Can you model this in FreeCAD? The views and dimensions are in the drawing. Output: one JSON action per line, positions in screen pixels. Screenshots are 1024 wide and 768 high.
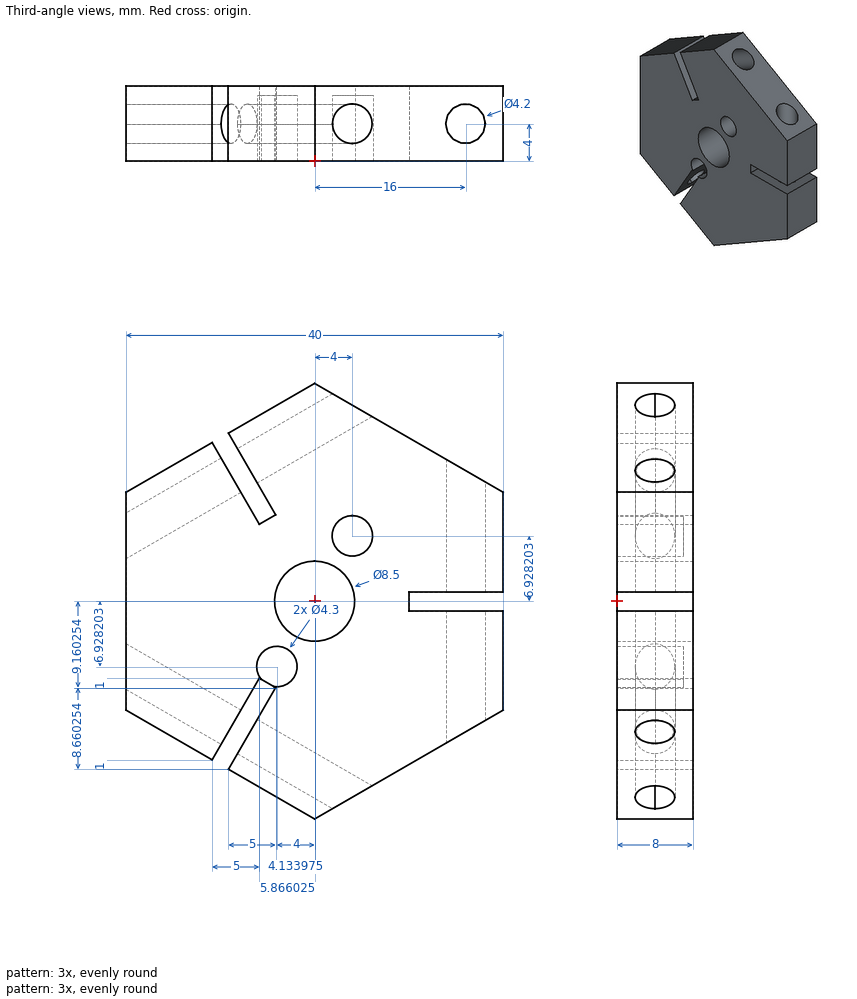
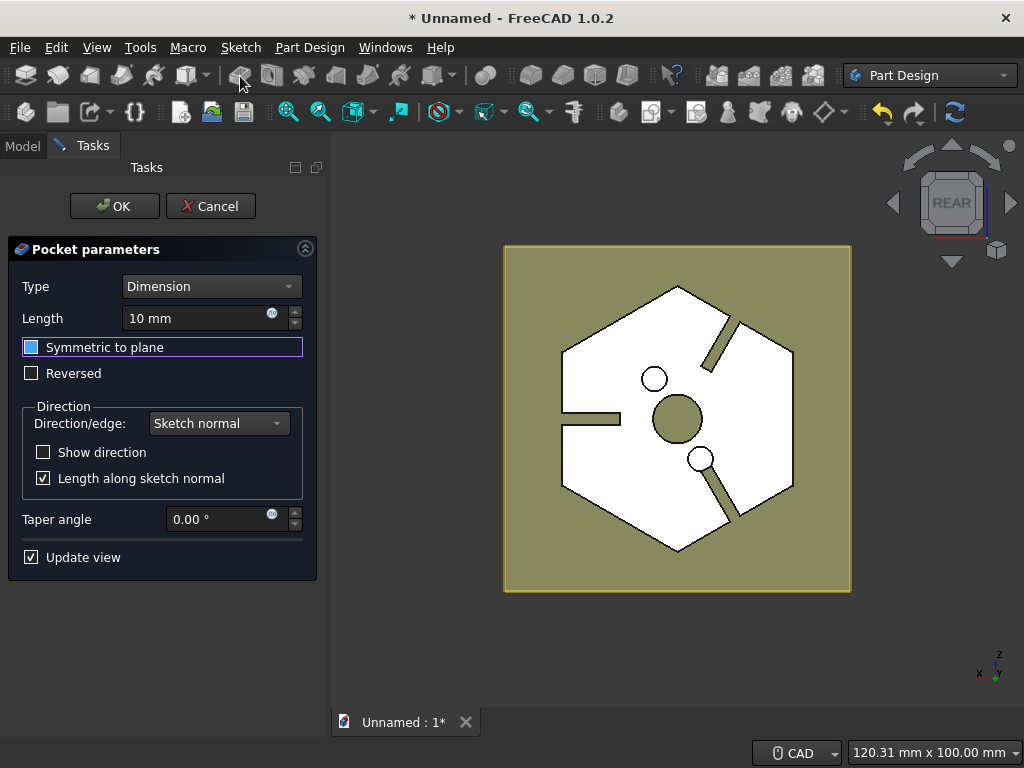
{"action": "left_click", "coordinate": [30, 373]}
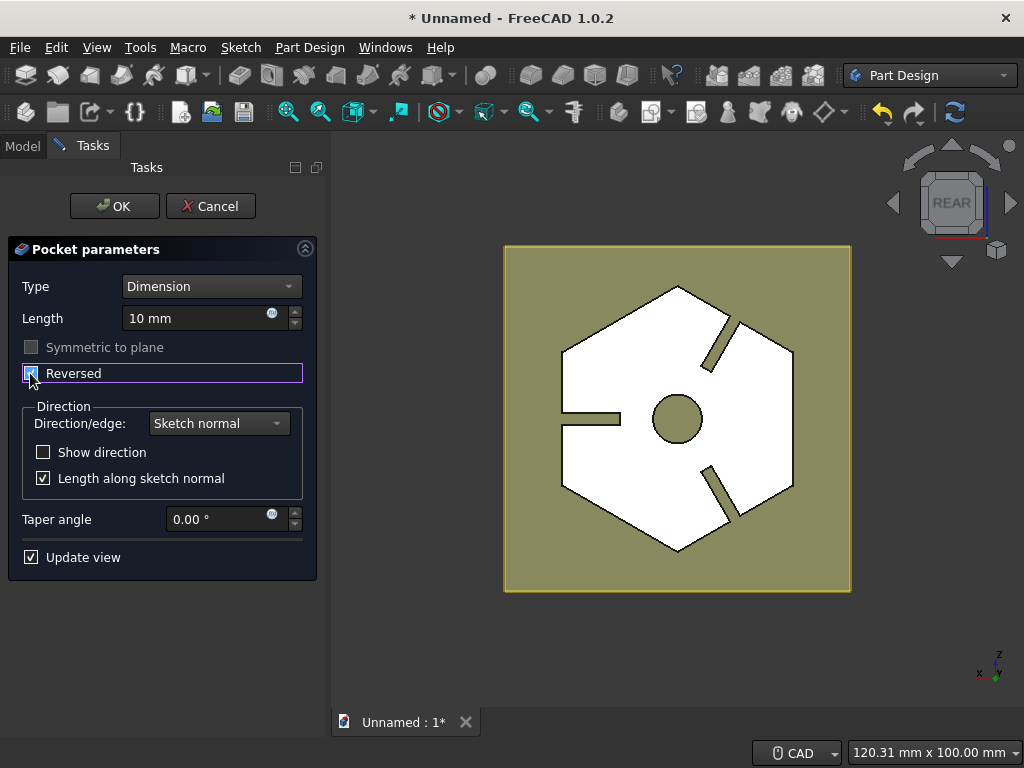
{"action": "left_click", "coordinate": [115, 206]}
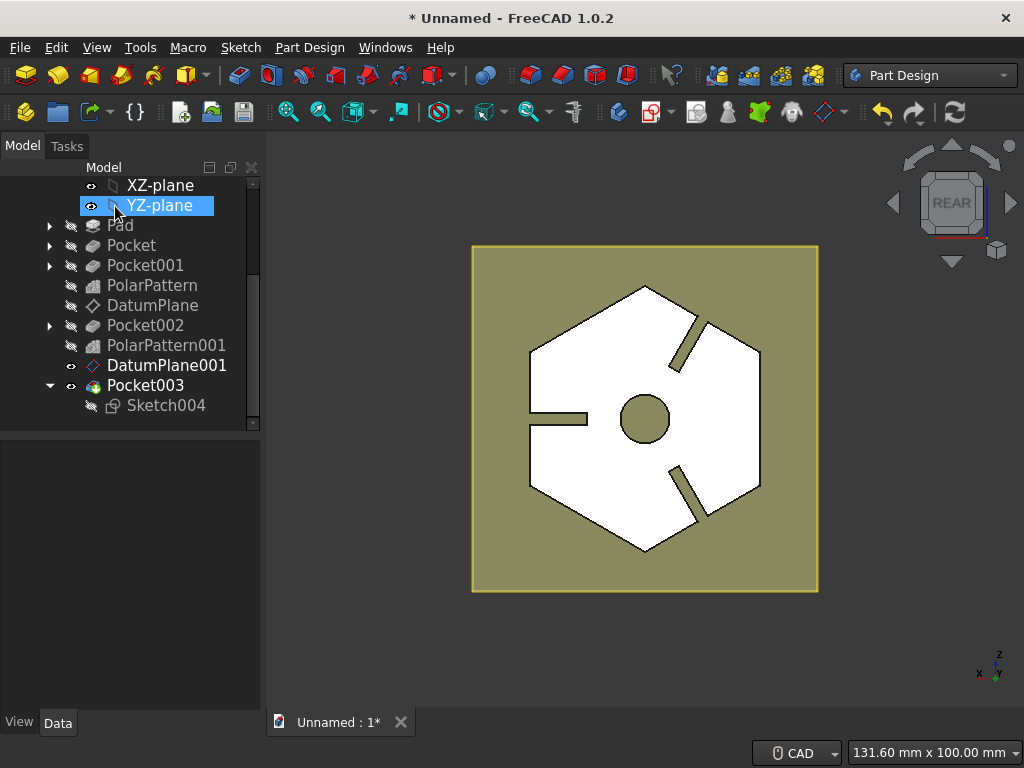
{"action": "left_click", "coordinate": [116, 366]}
{"action": "key", "text": "space"}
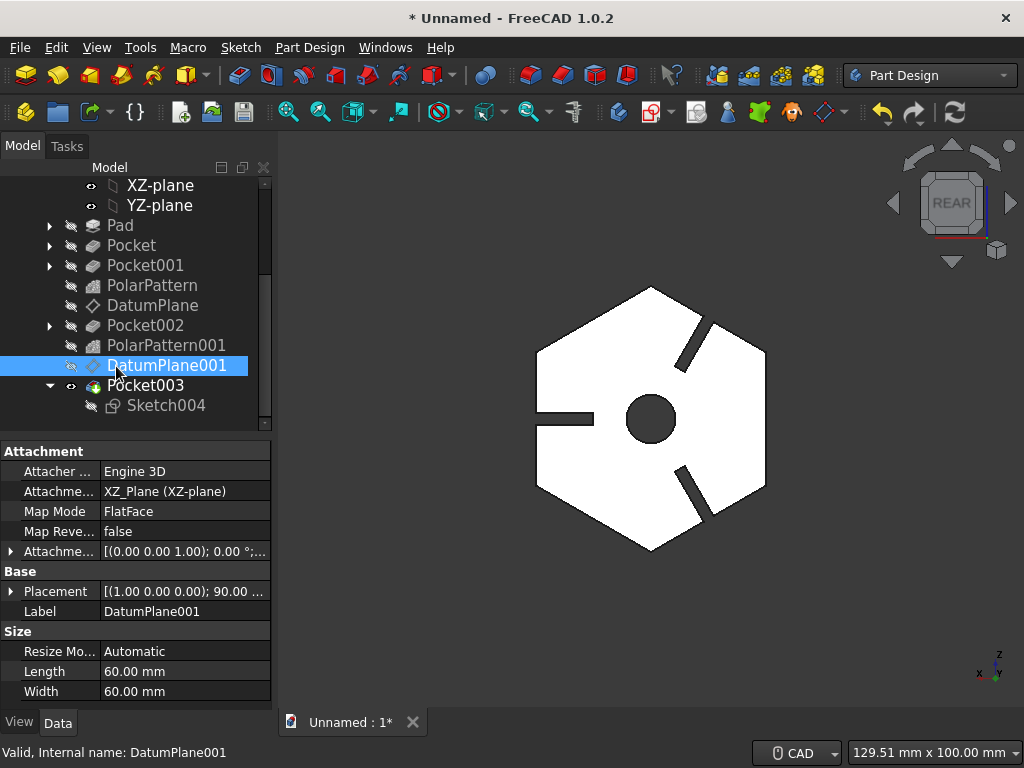
{"action": "key", "text": "0"}